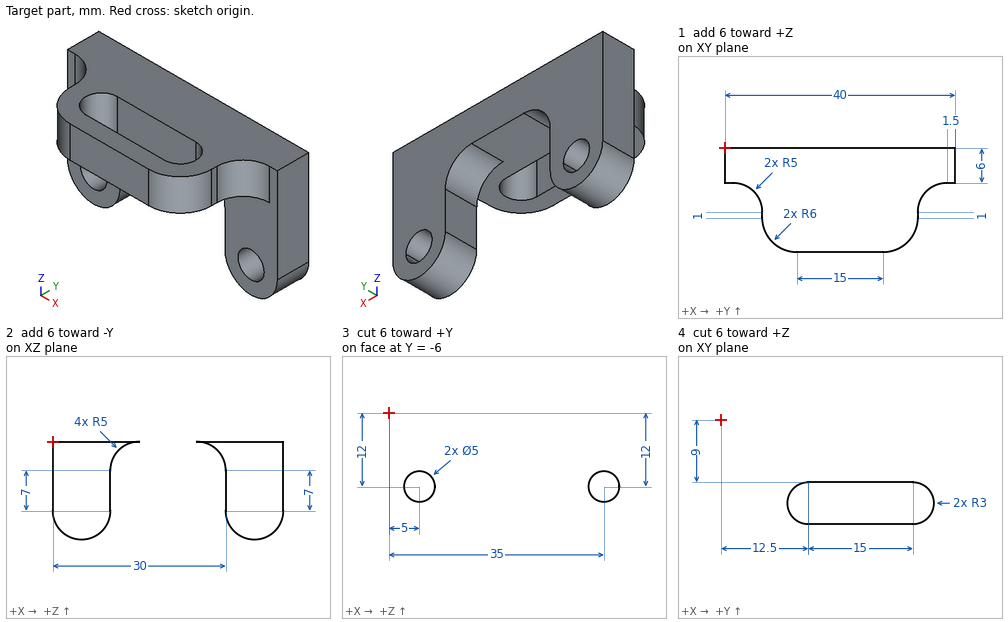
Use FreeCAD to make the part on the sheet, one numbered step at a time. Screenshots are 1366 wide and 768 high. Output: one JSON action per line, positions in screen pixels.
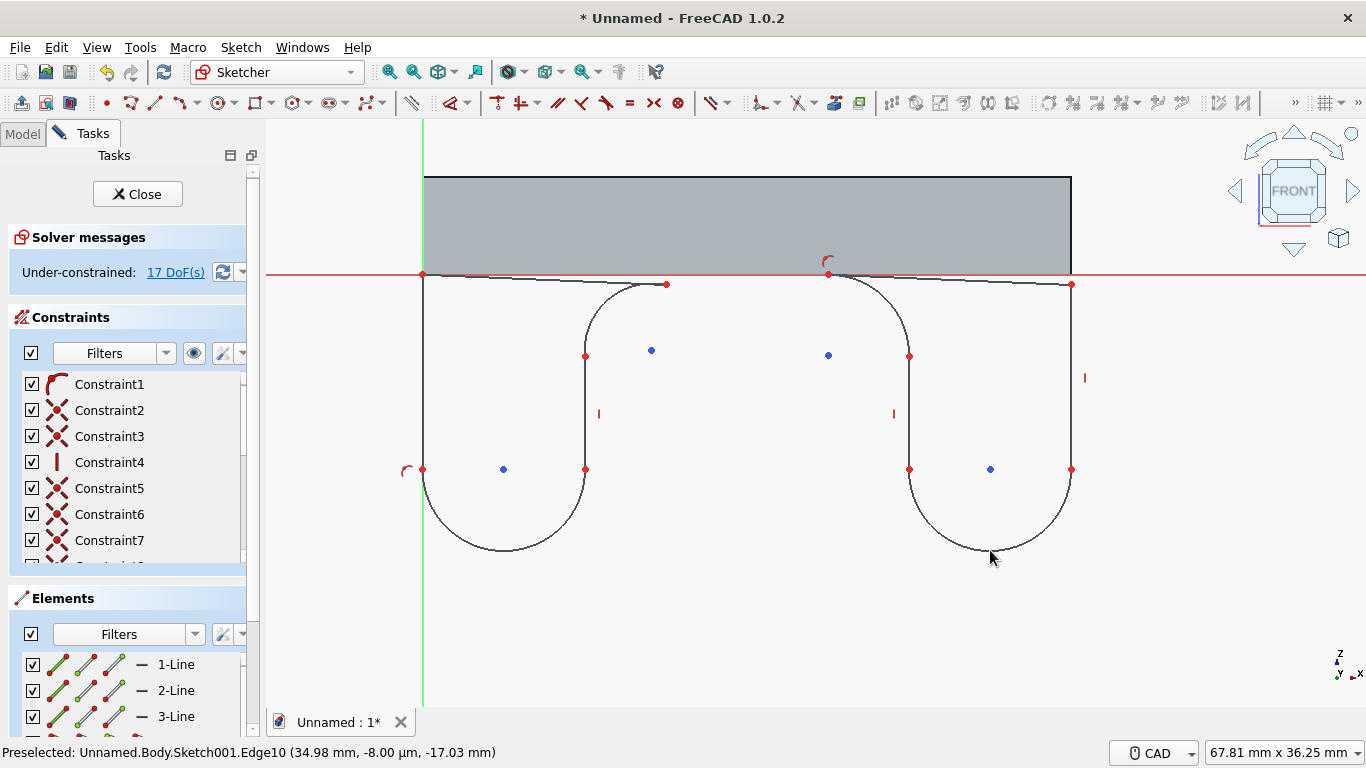
{"action": "left_click", "coordinate": [423, 411]}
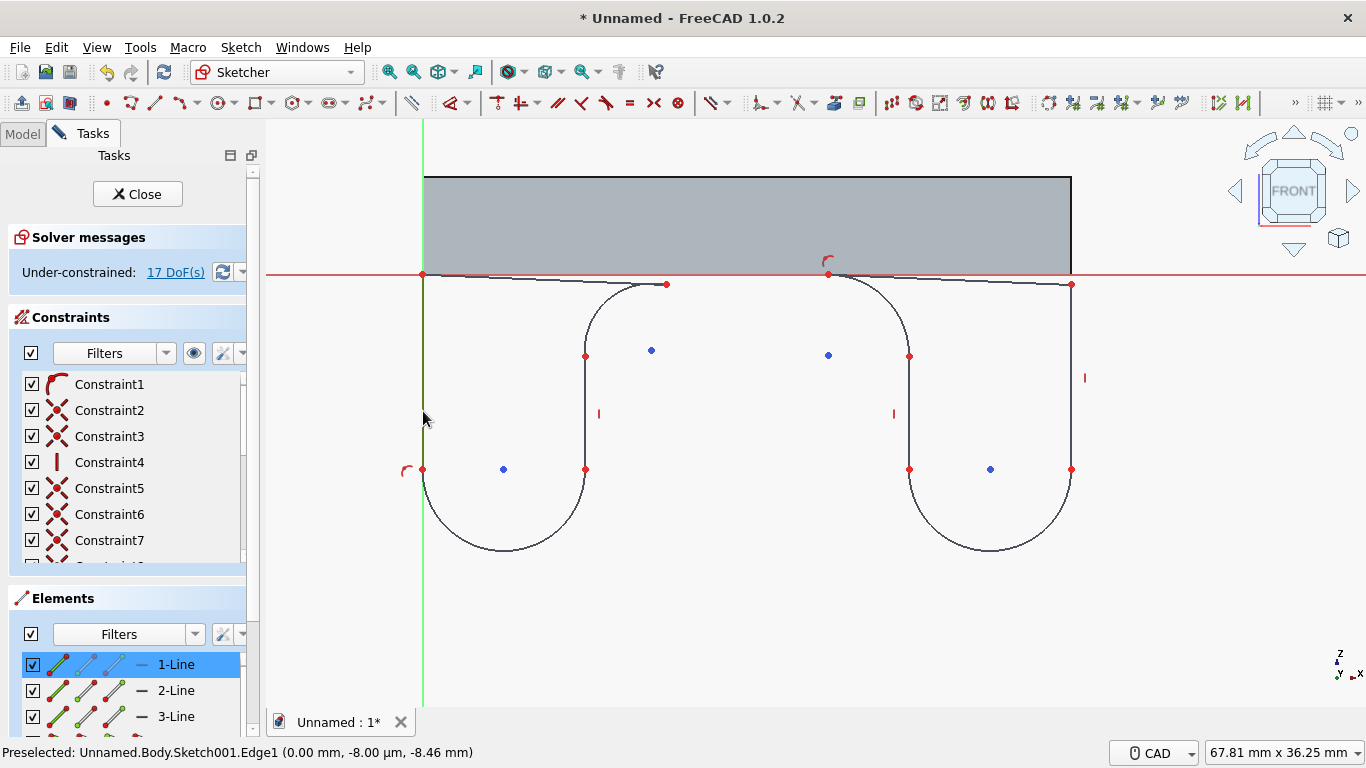
{"action": "left_click", "coordinate": [456, 536]}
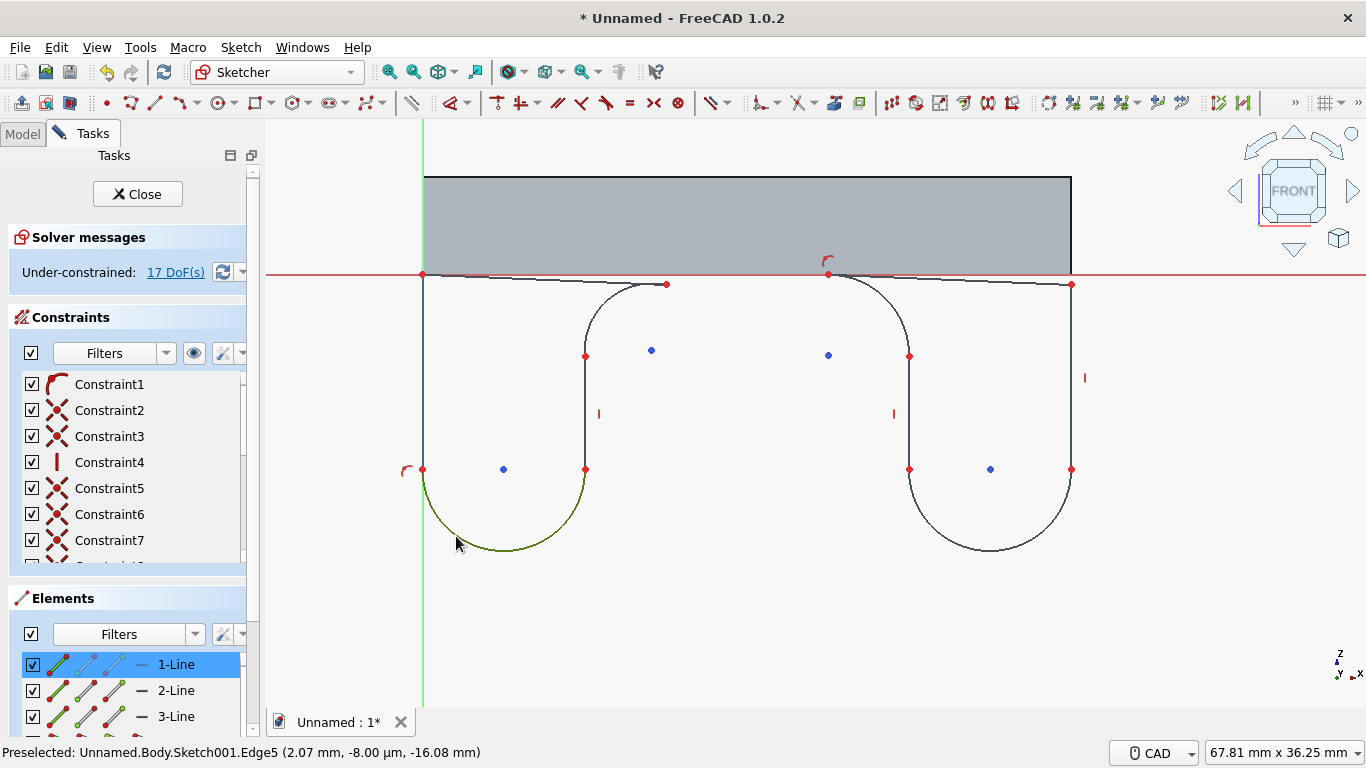
{"action": "key", "text": "t"}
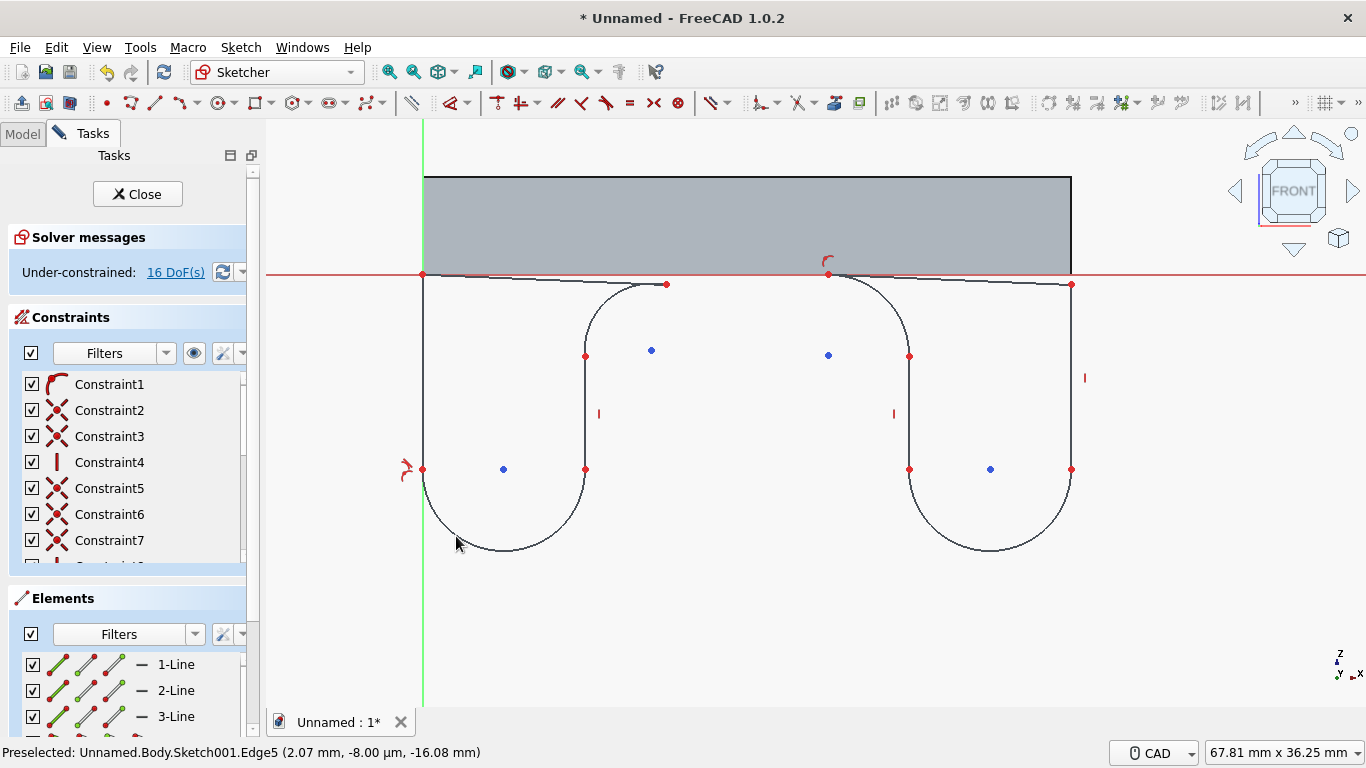
{"action": "left_click", "coordinate": [496, 278]}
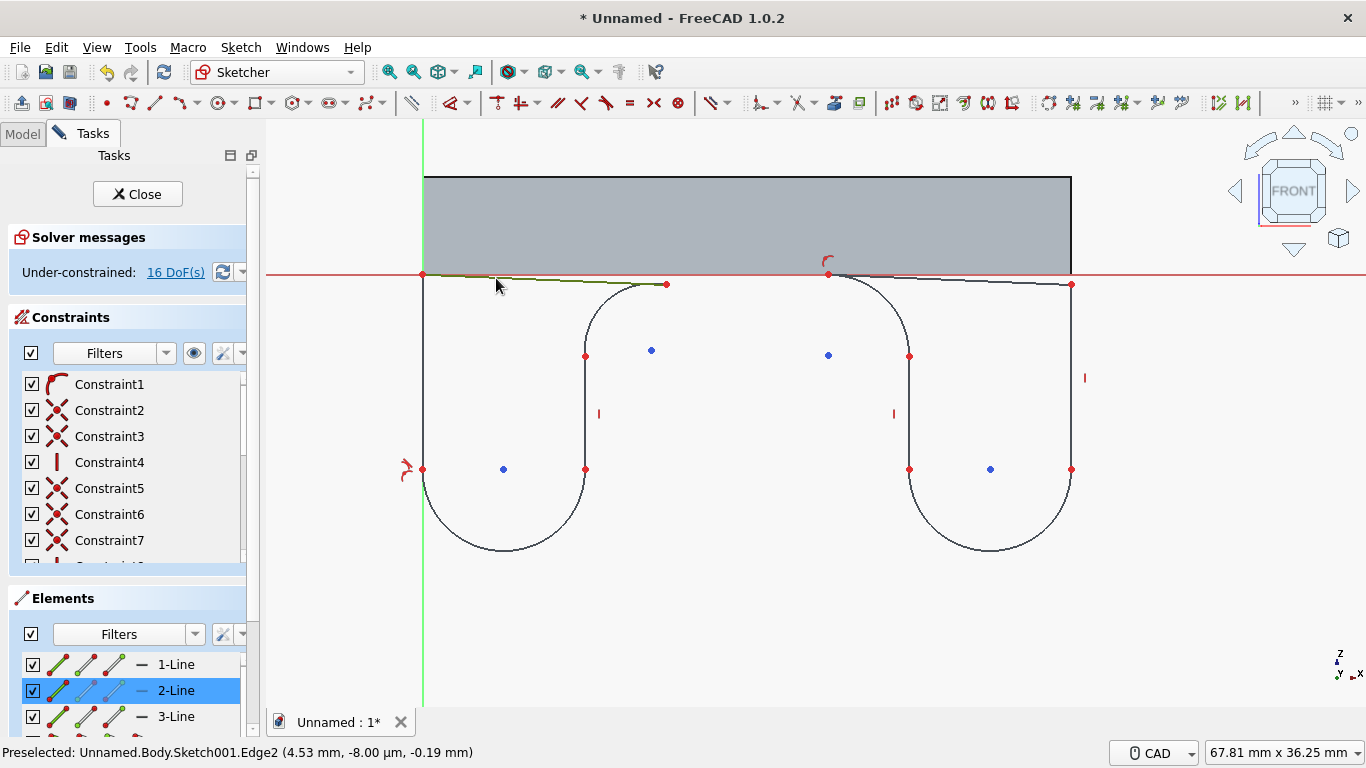
{"action": "left_click", "coordinate": [592, 320]}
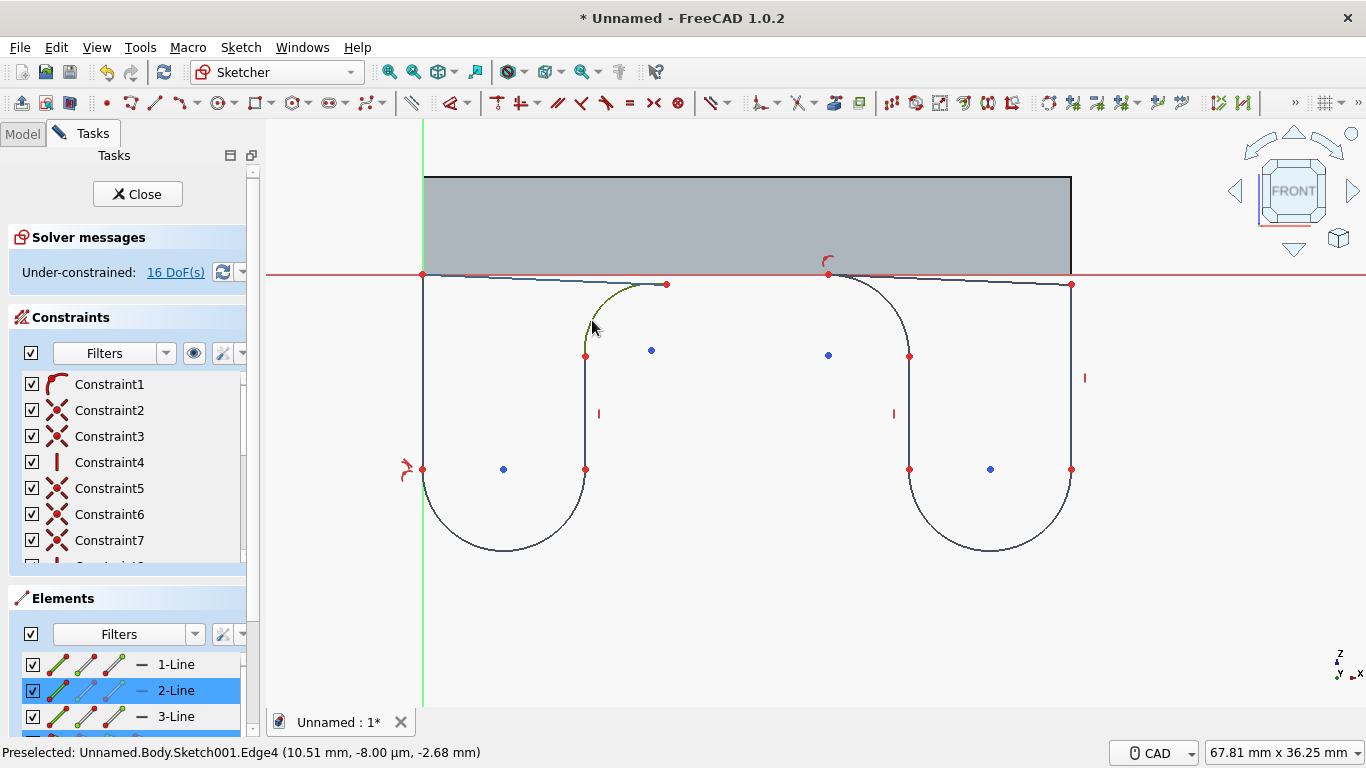
{"action": "key", "text": "t"}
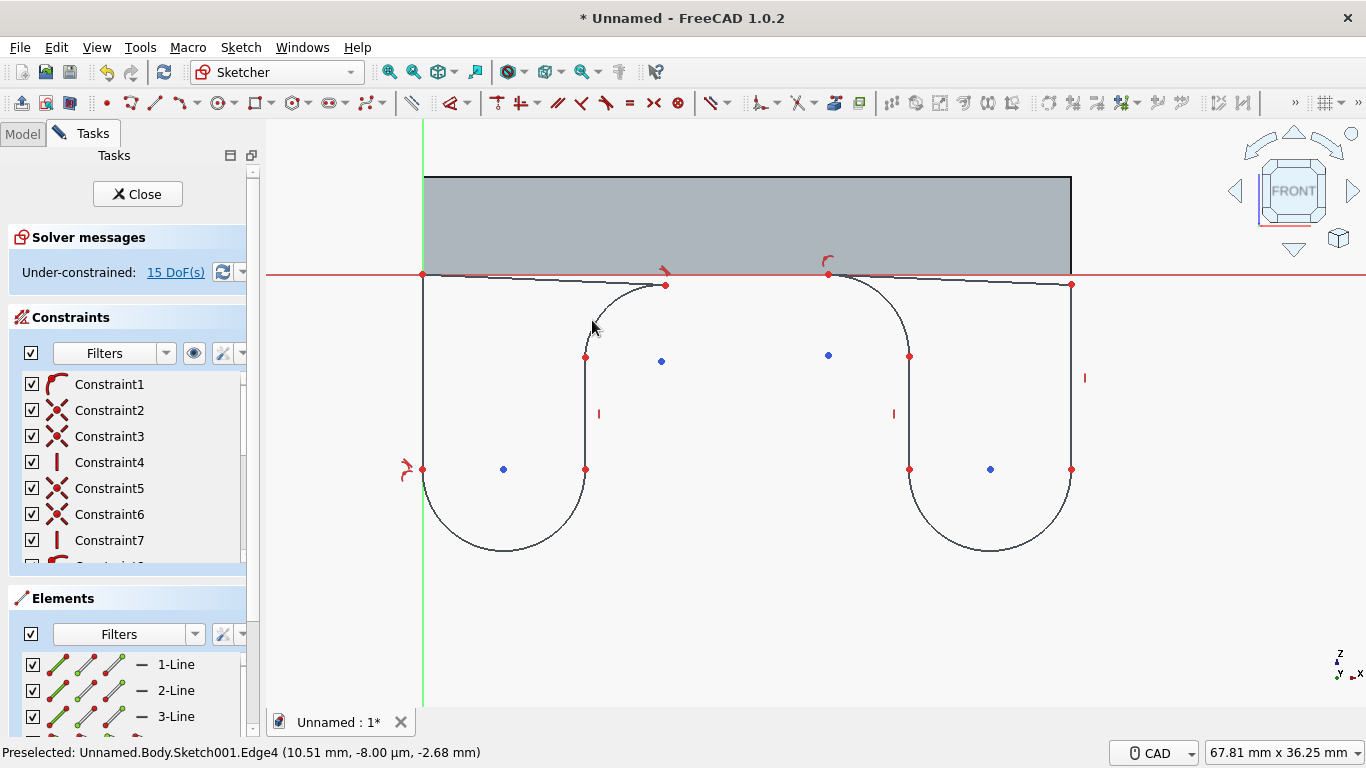
{"action": "left_click", "coordinate": [585, 391]}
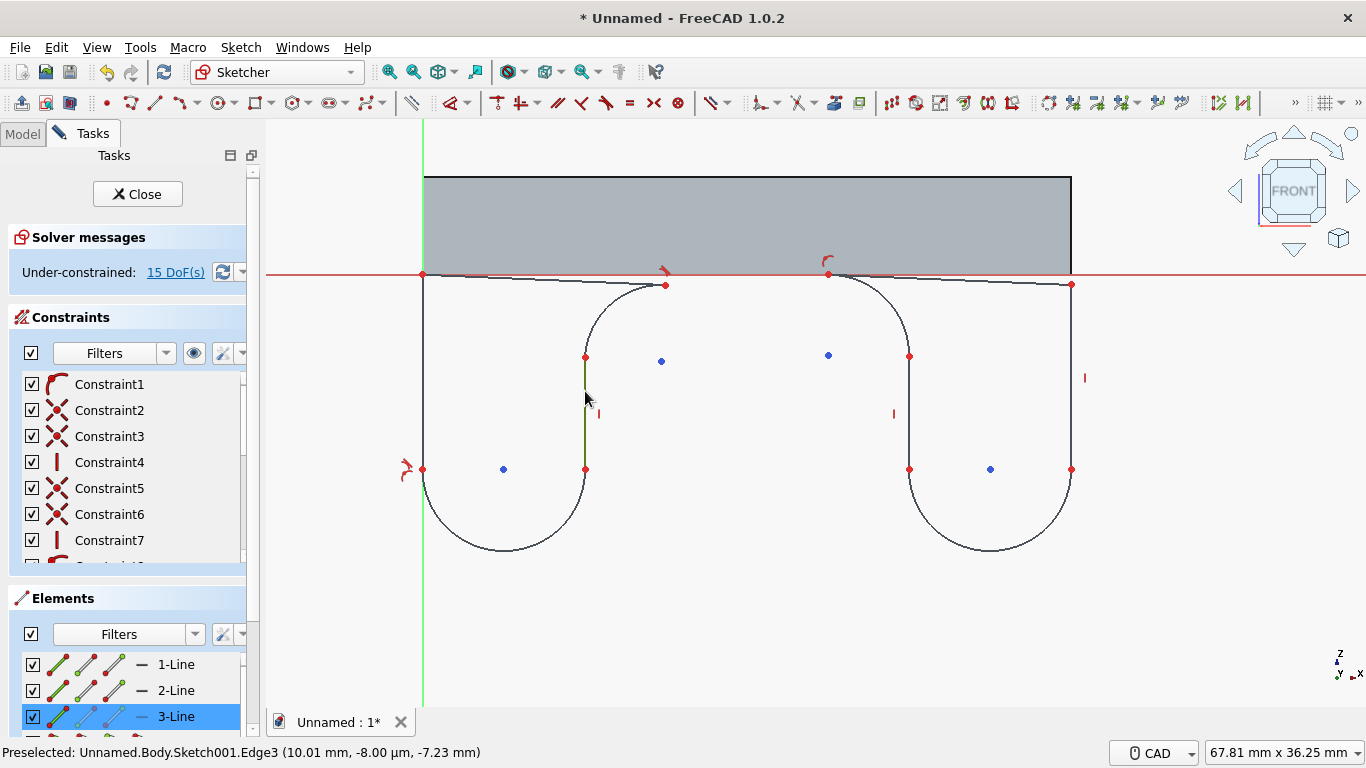
{"action": "left_click", "coordinate": [595, 323]}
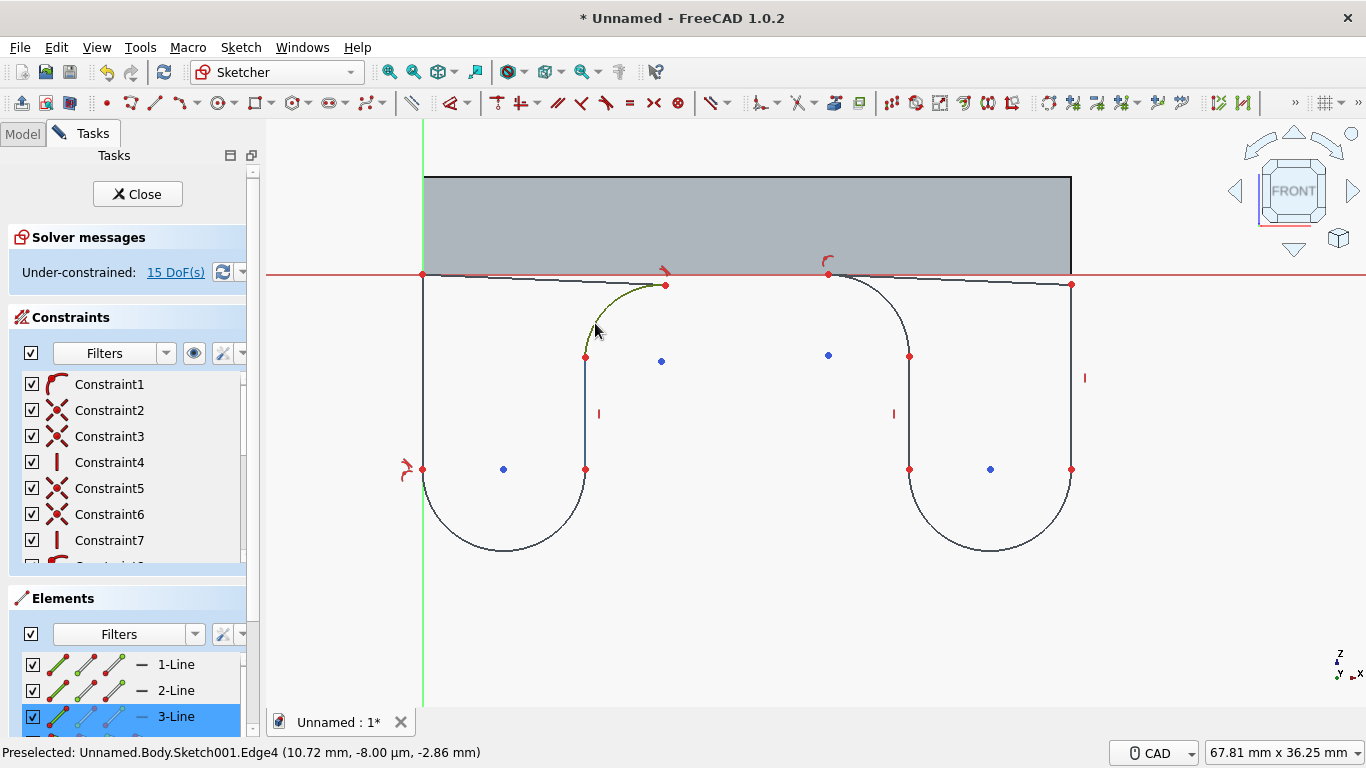
{"action": "left_click", "coordinate": [606, 104]}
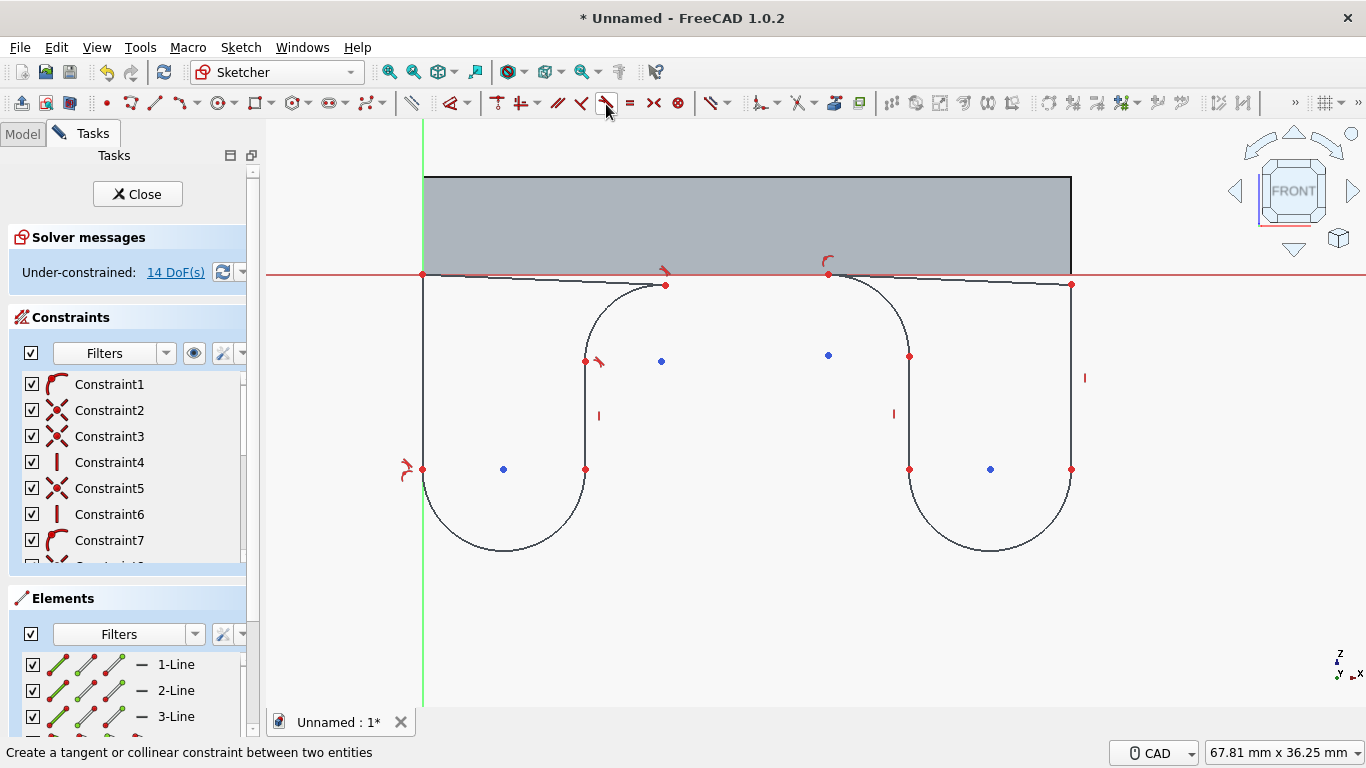
{"action": "left_click", "coordinate": [585, 394]}